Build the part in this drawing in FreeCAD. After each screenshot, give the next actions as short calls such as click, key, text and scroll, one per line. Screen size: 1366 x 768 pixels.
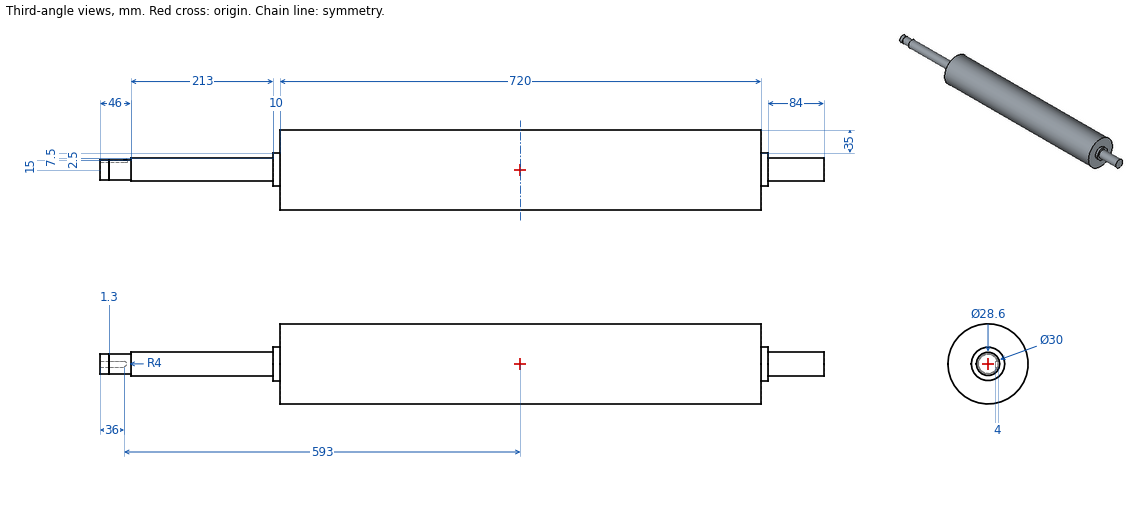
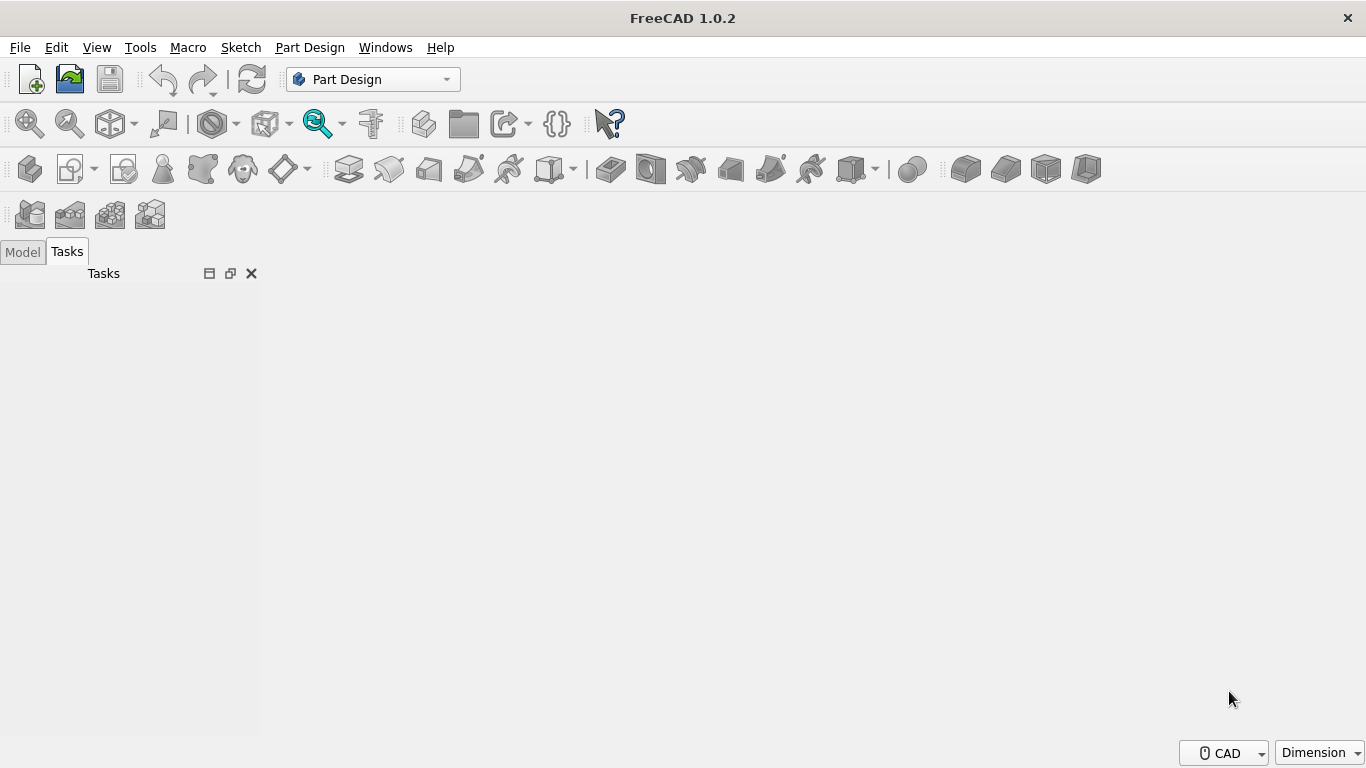
click(30, 80)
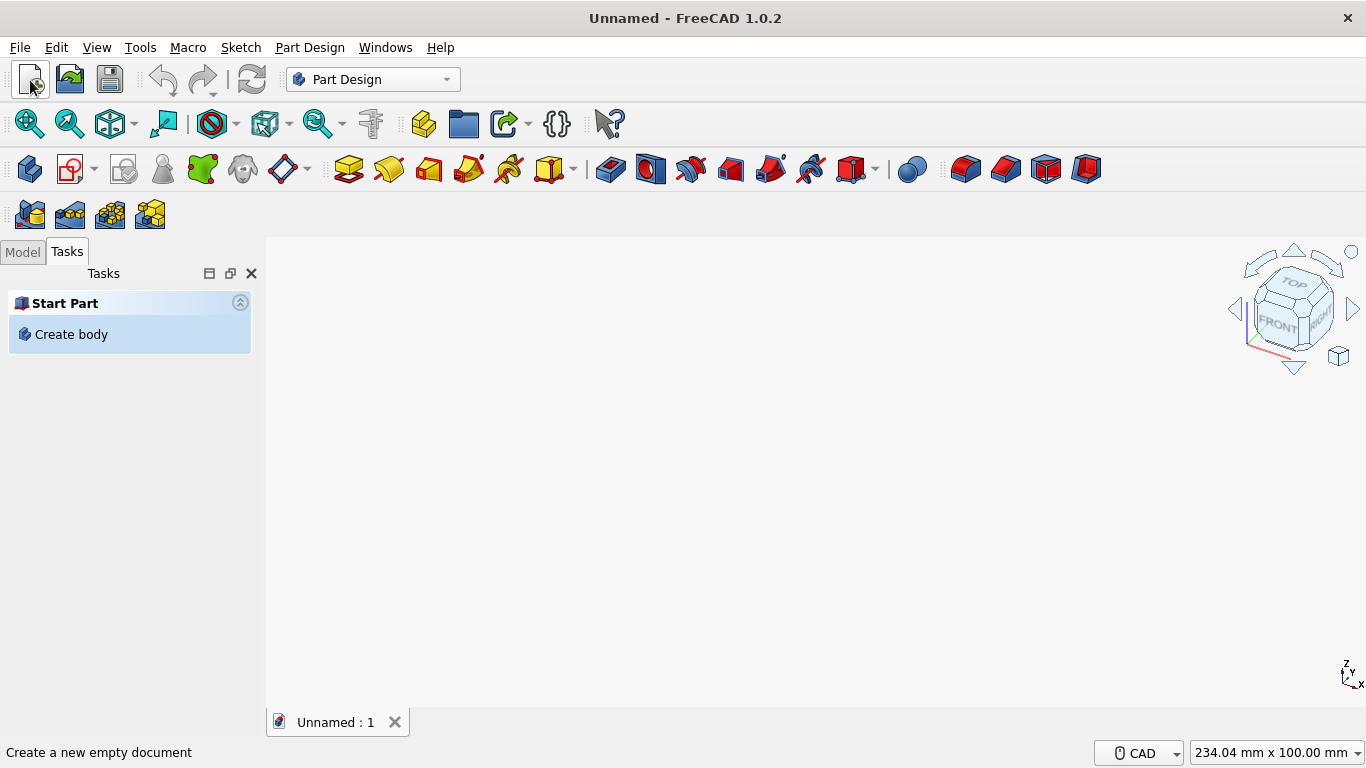
click(70, 170)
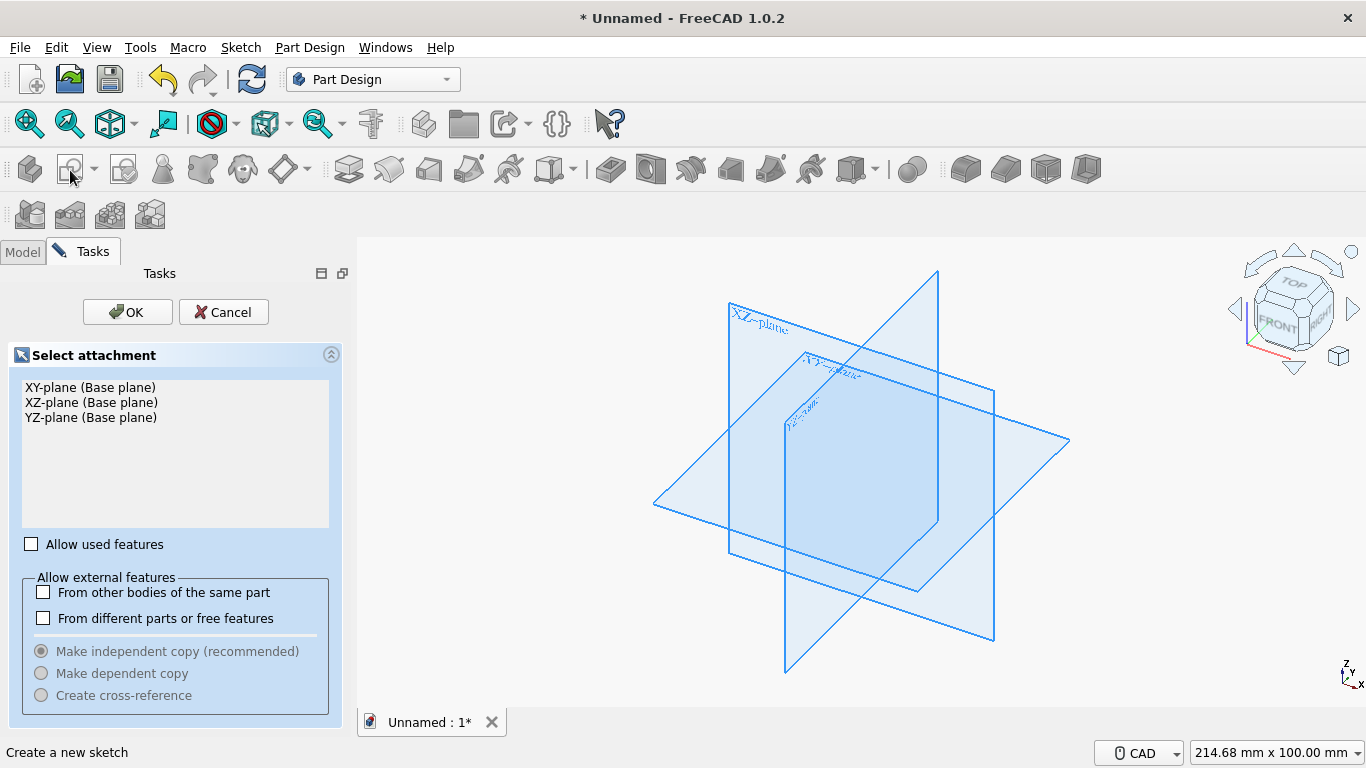
click(82, 388)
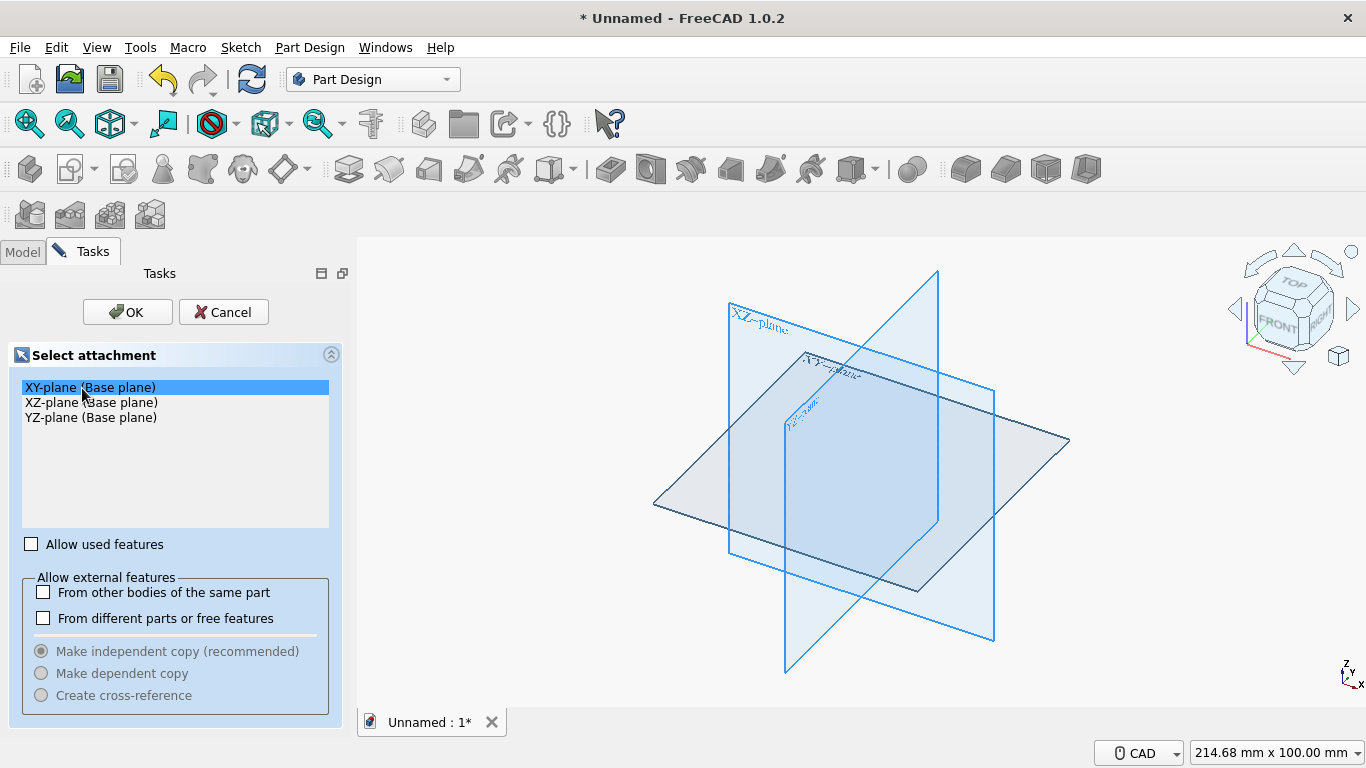
click(128, 312)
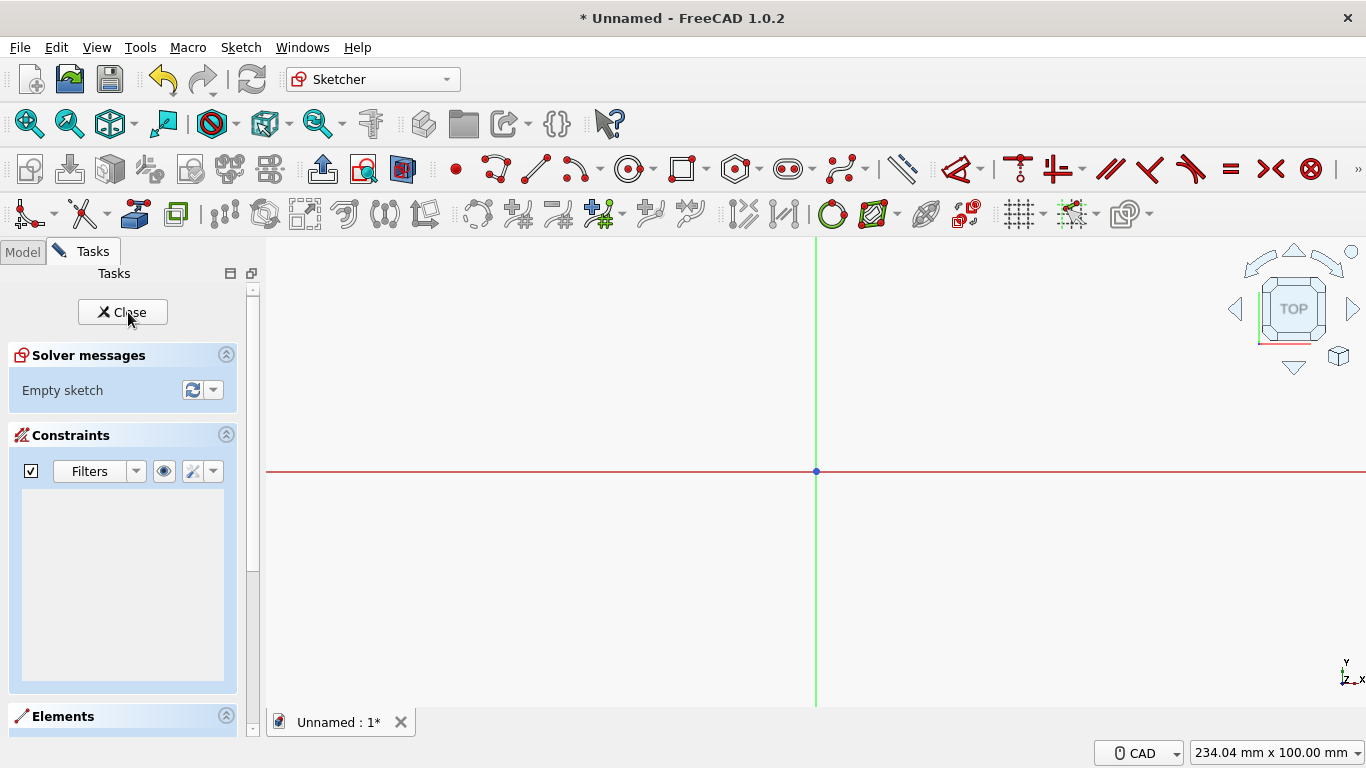
scroll(801, 494, down, 10)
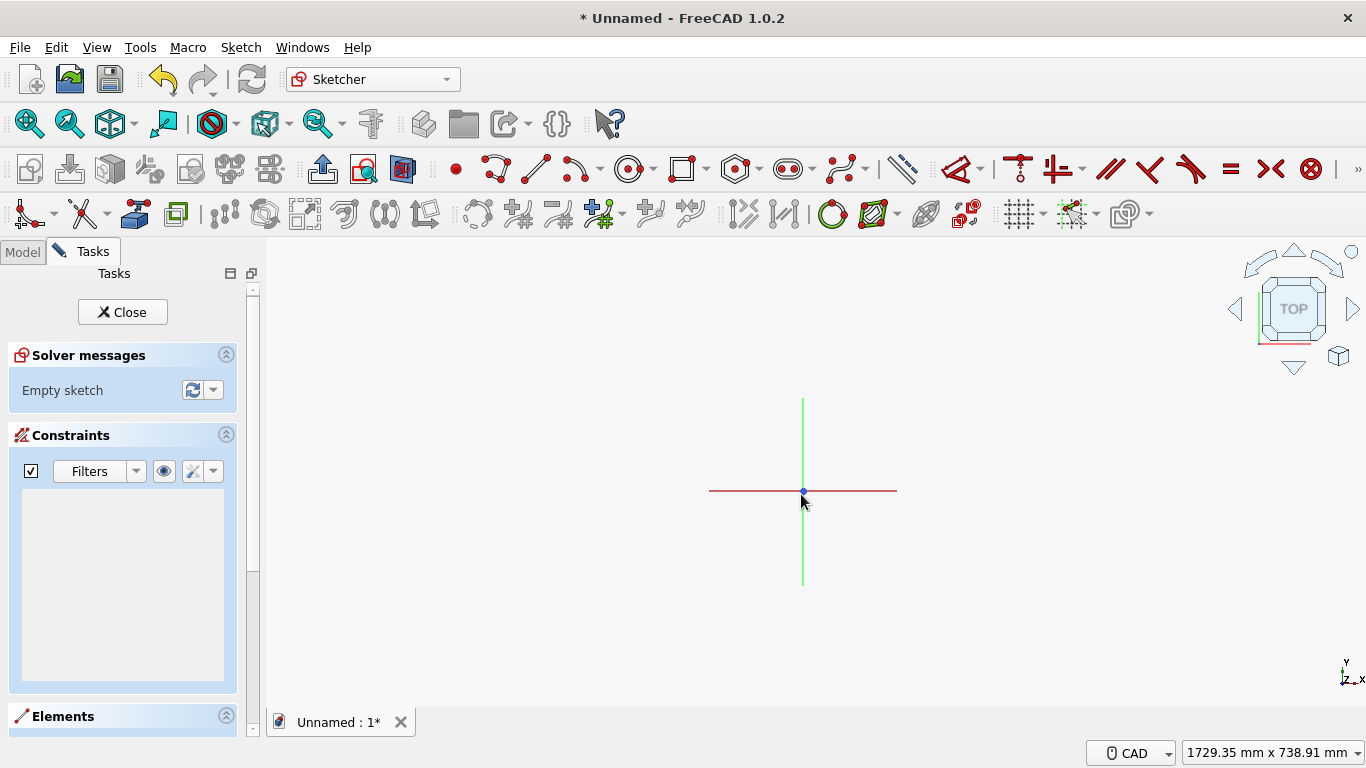
key(g)
key(m)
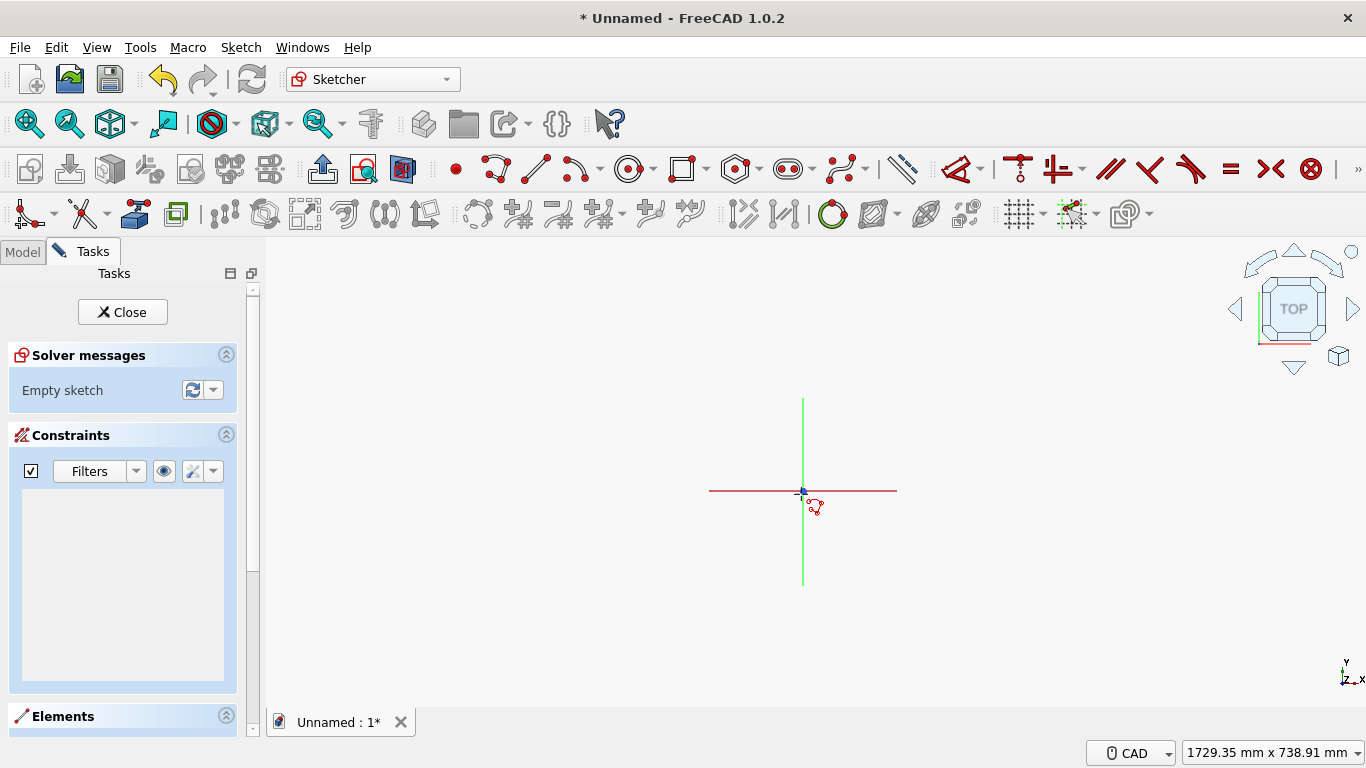
click(574, 476)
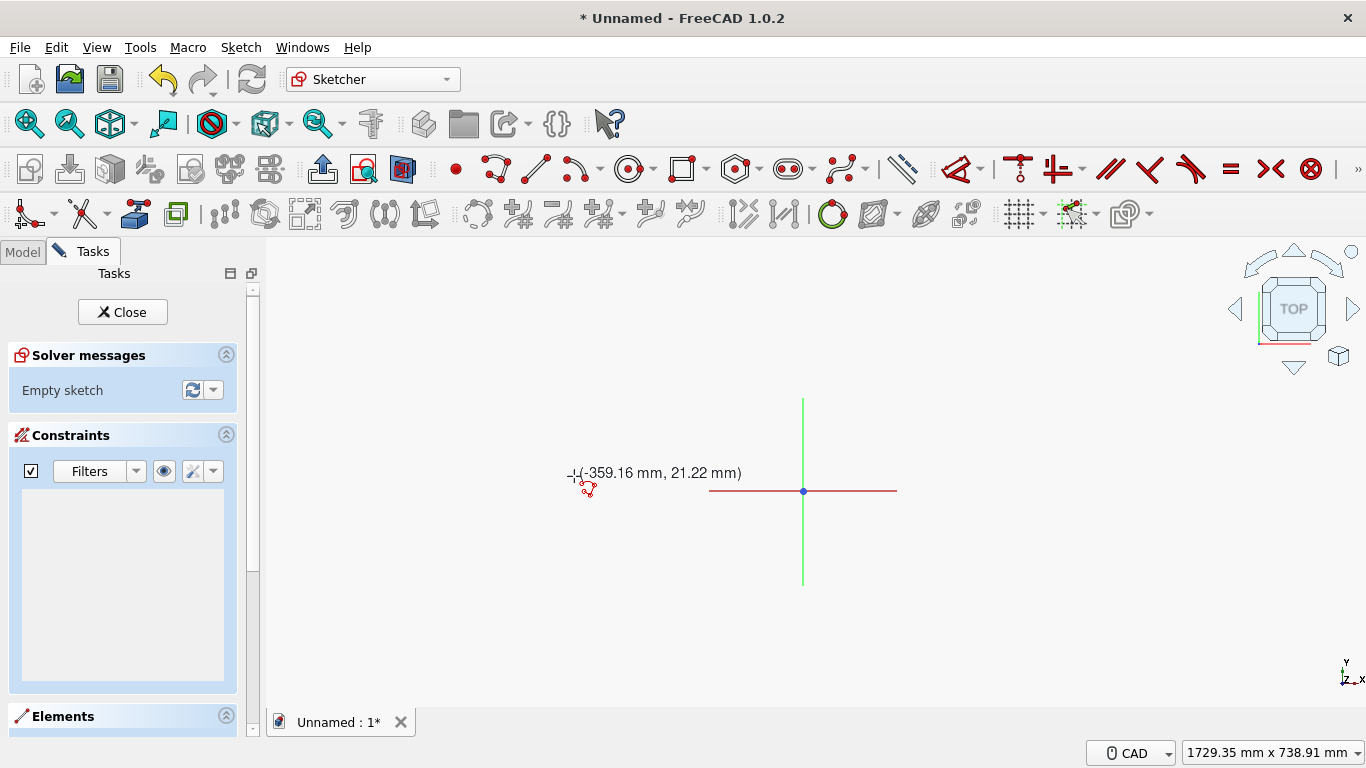
scroll(568, 476, up, 5)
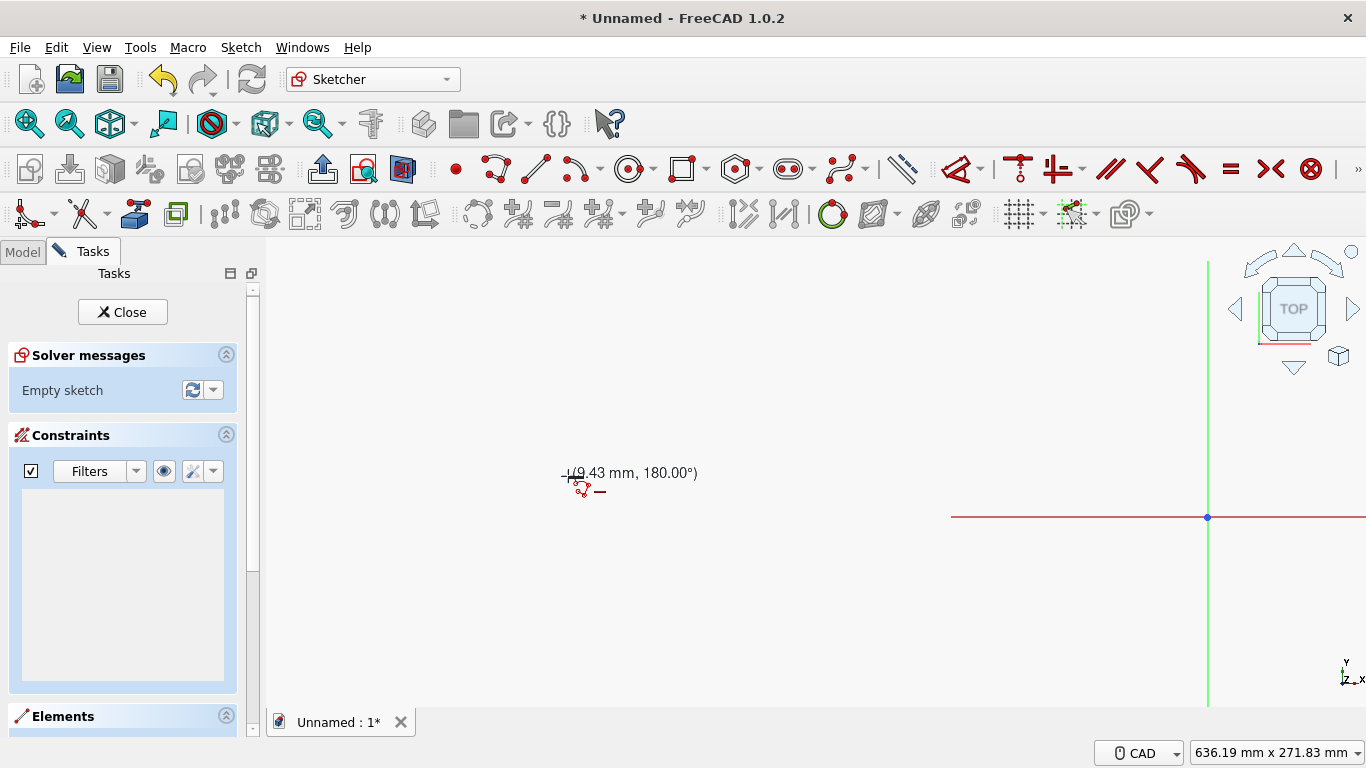
click(568, 475)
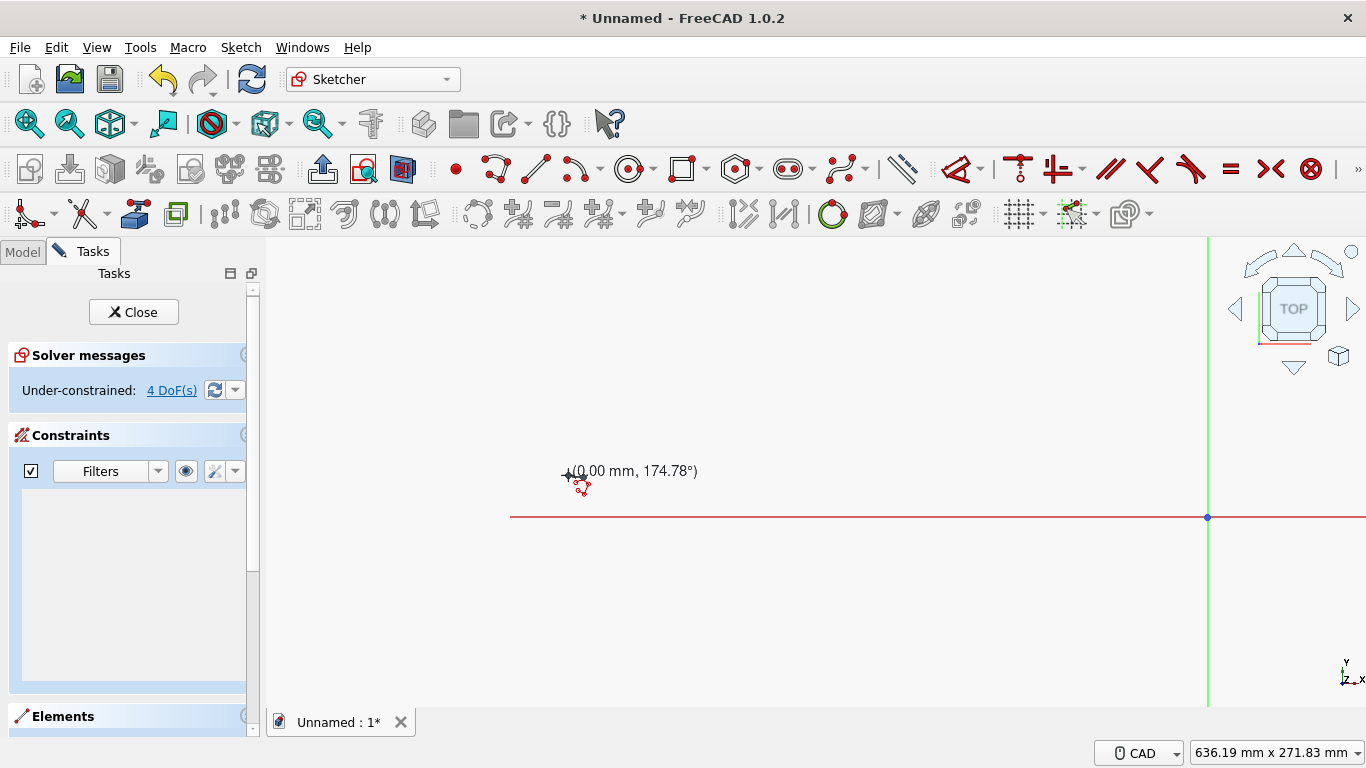
scroll(568, 487, up, 2)